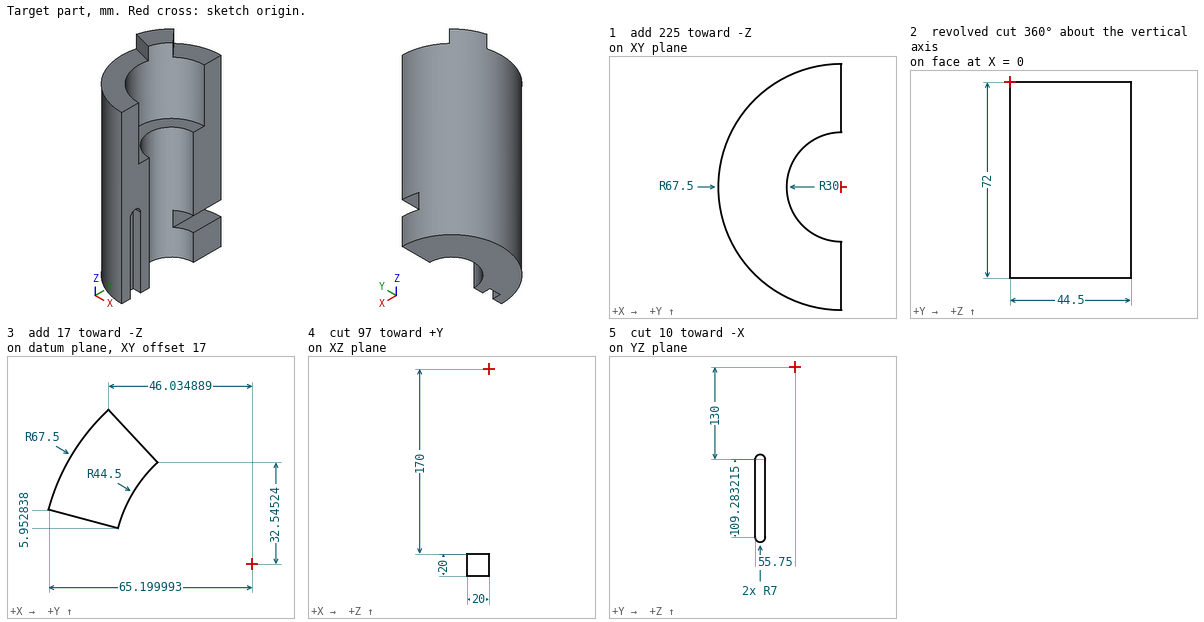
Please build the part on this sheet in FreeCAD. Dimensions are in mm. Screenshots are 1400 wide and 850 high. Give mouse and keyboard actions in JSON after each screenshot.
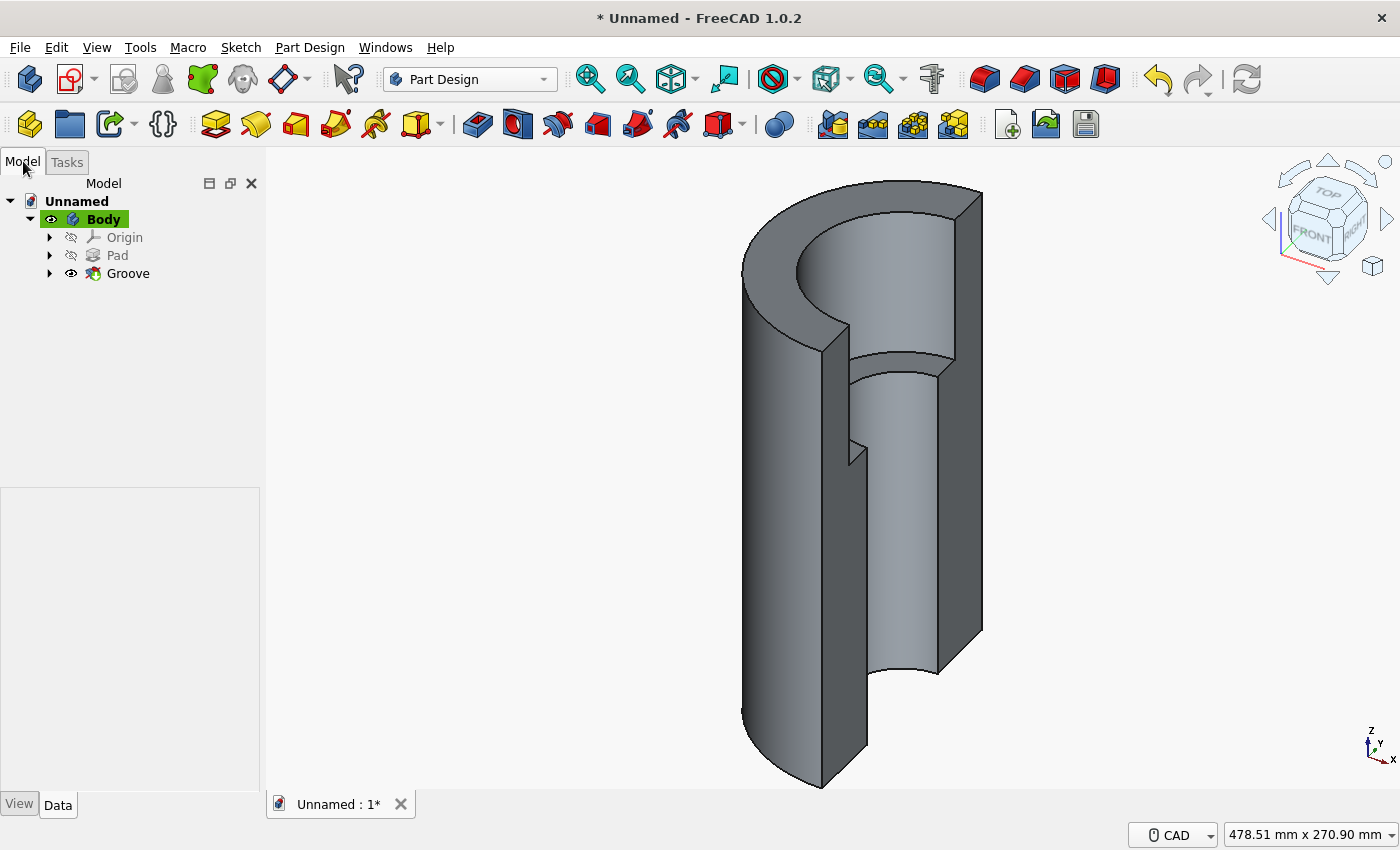
{"action": "left_click", "coordinate": [50, 237]}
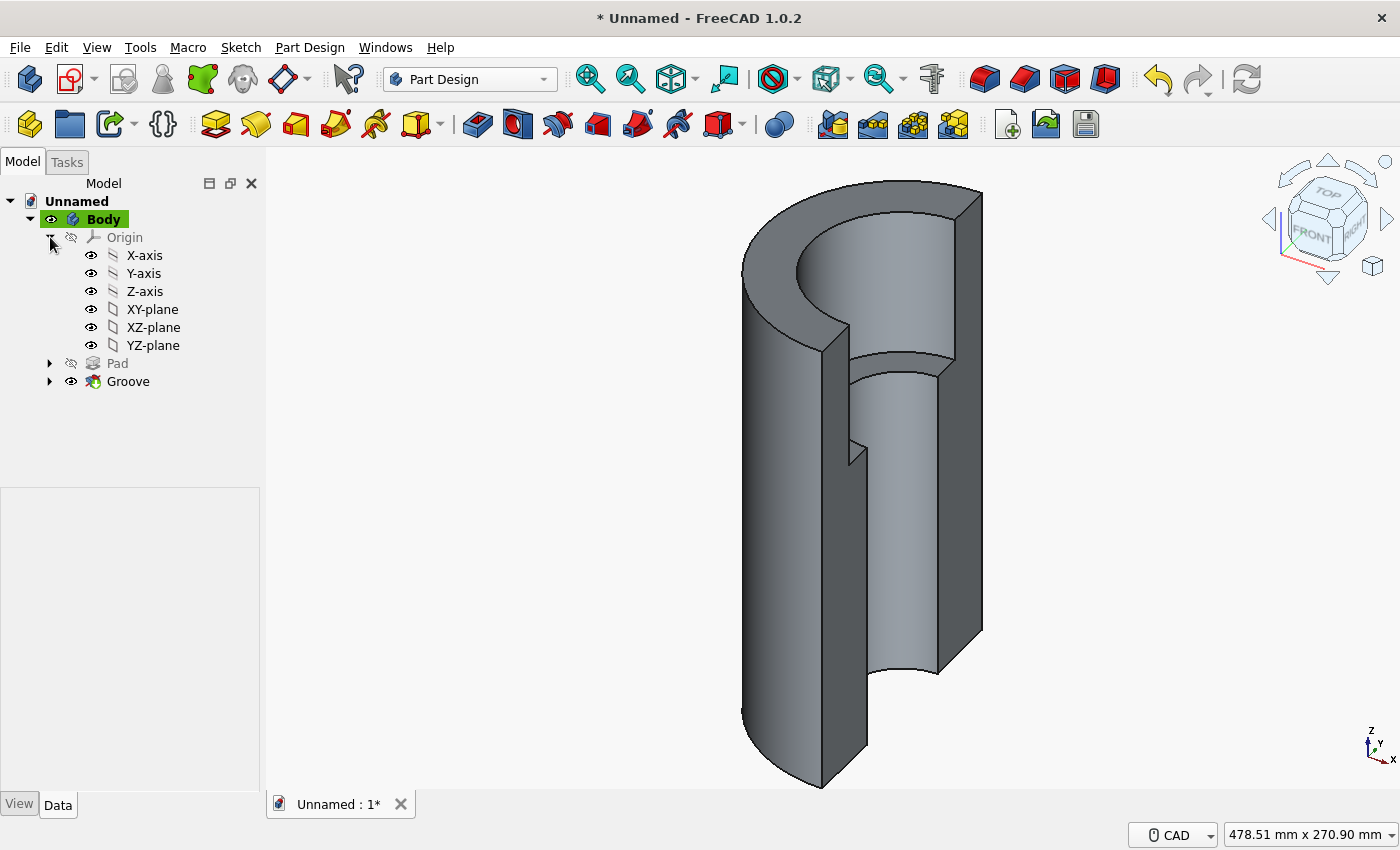
{"action": "left_click", "coordinate": [136, 309]}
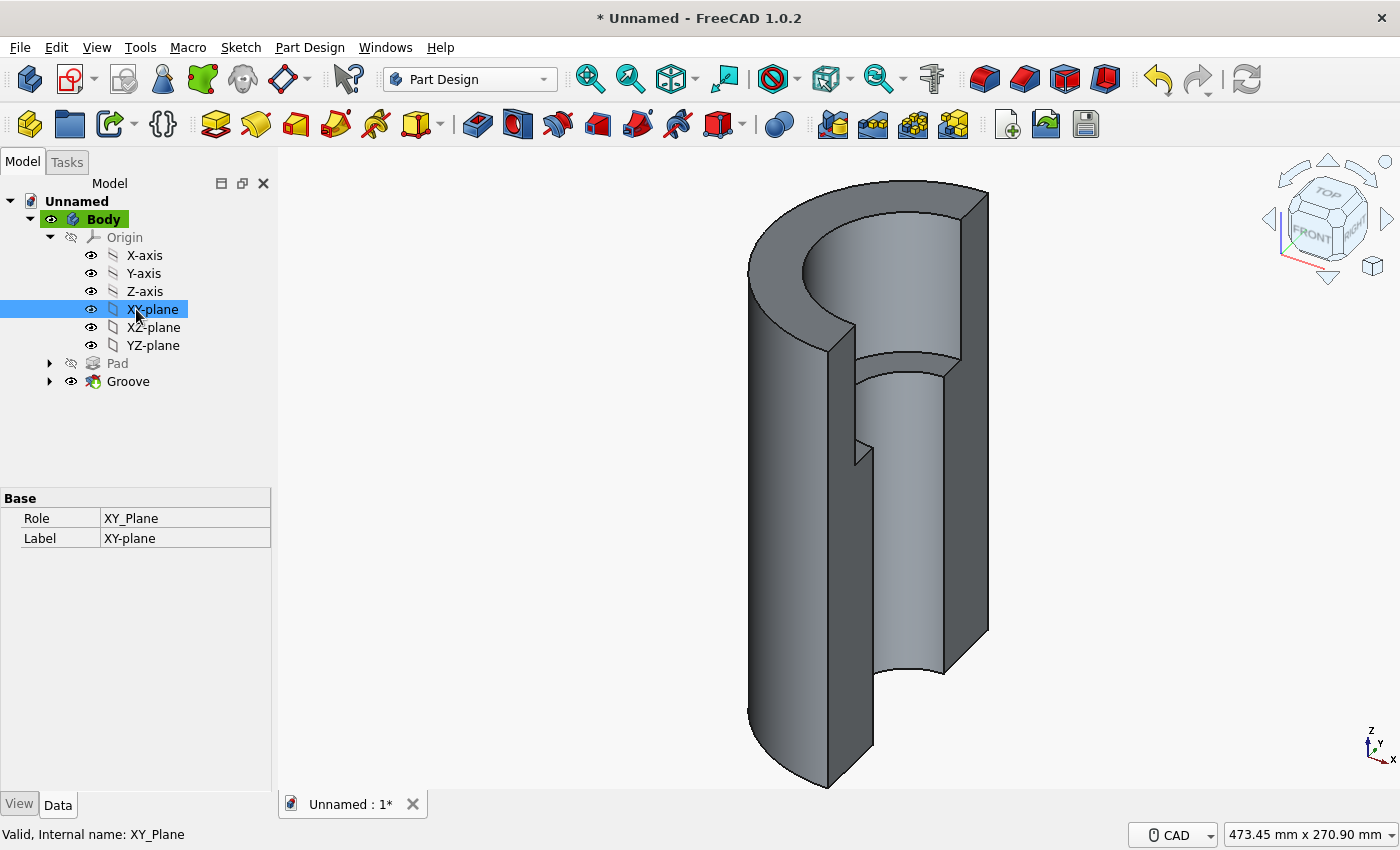
{"action": "left_click", "coordinate": [284, 80]}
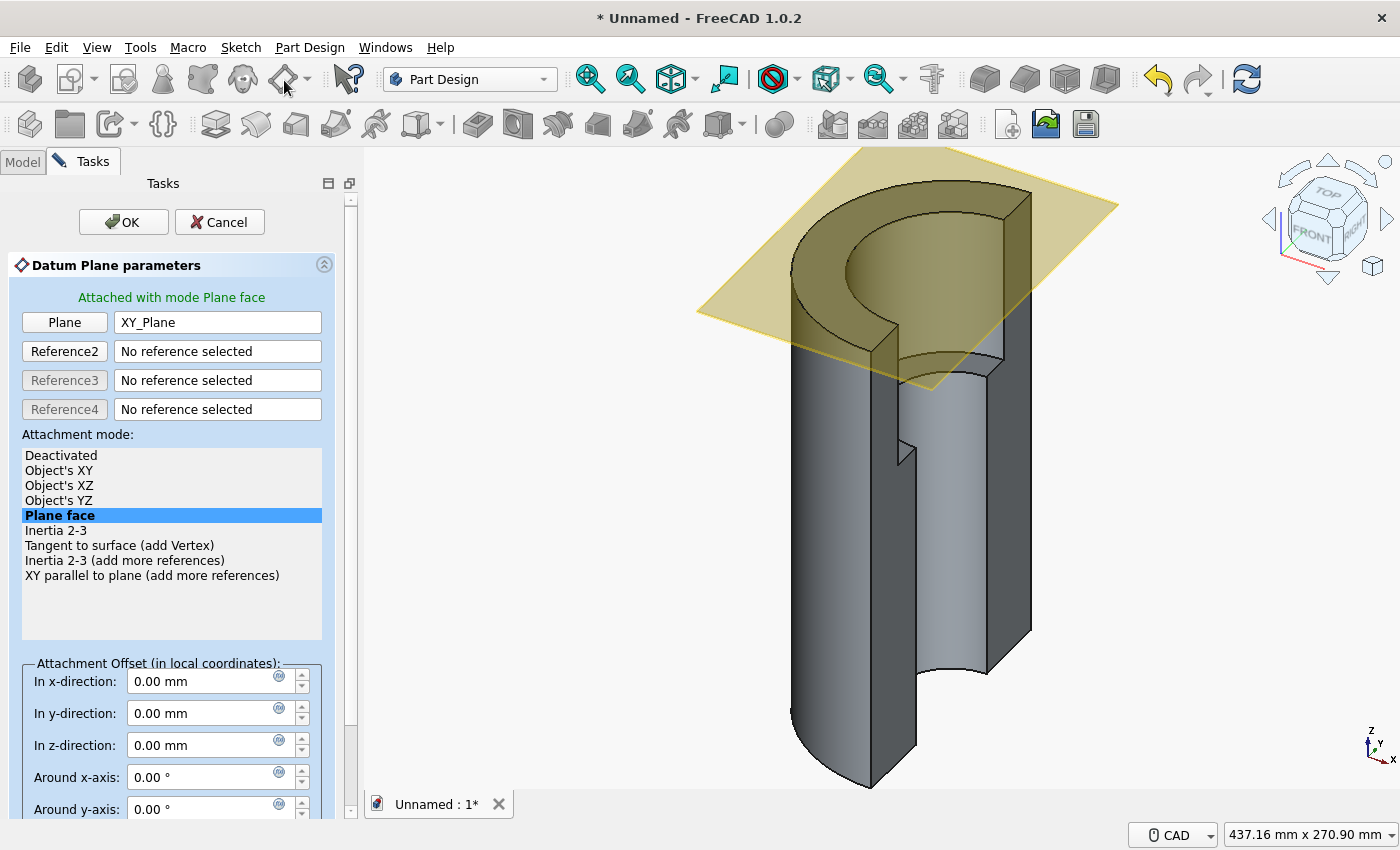
{"action": "triple_click", "coordinate": [210, 745]}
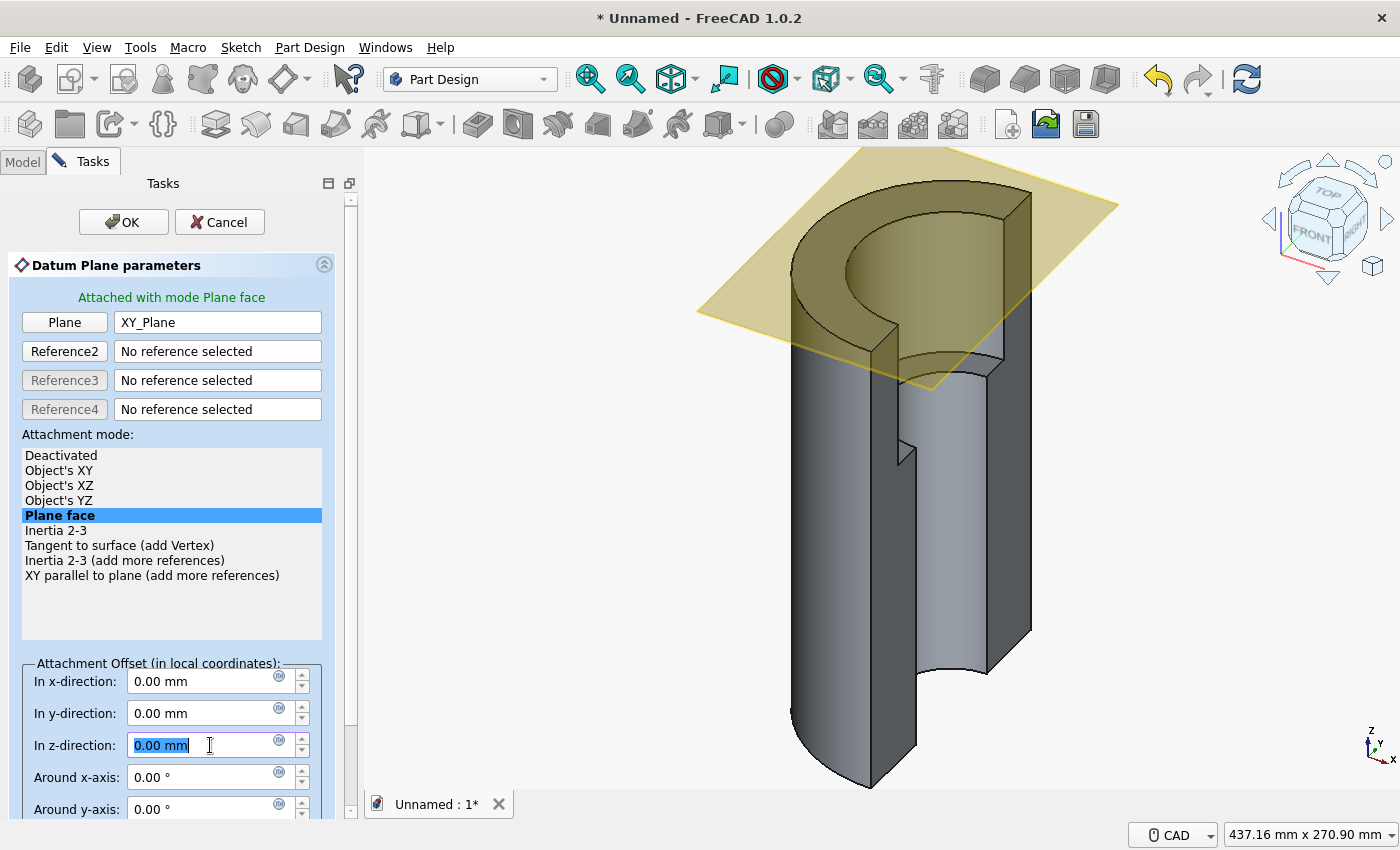
{"action": "type", "text": "17"}
{"action": "key", "text": "Tab"}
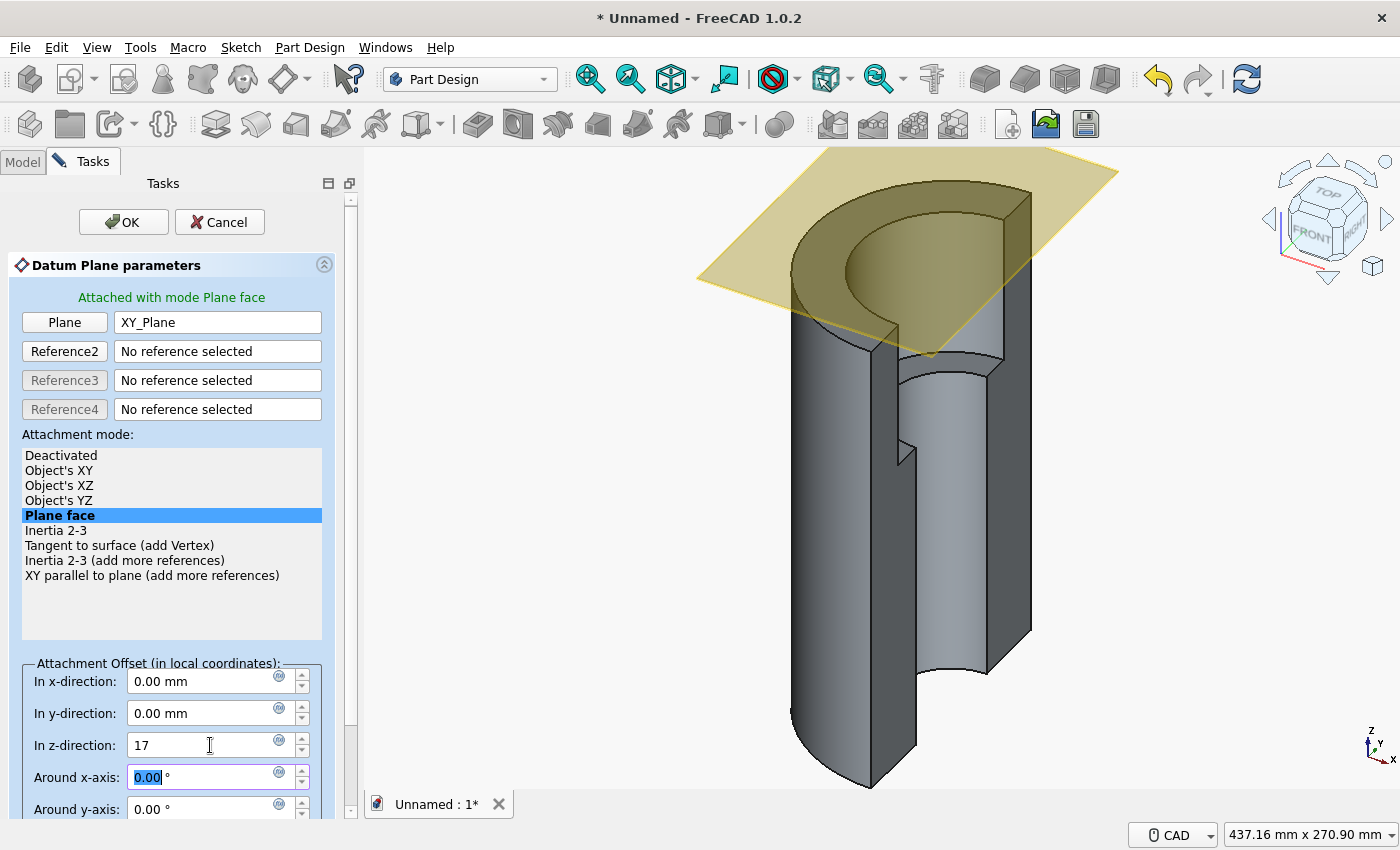
{"action": "left_click", "coordinate": [124, 222]}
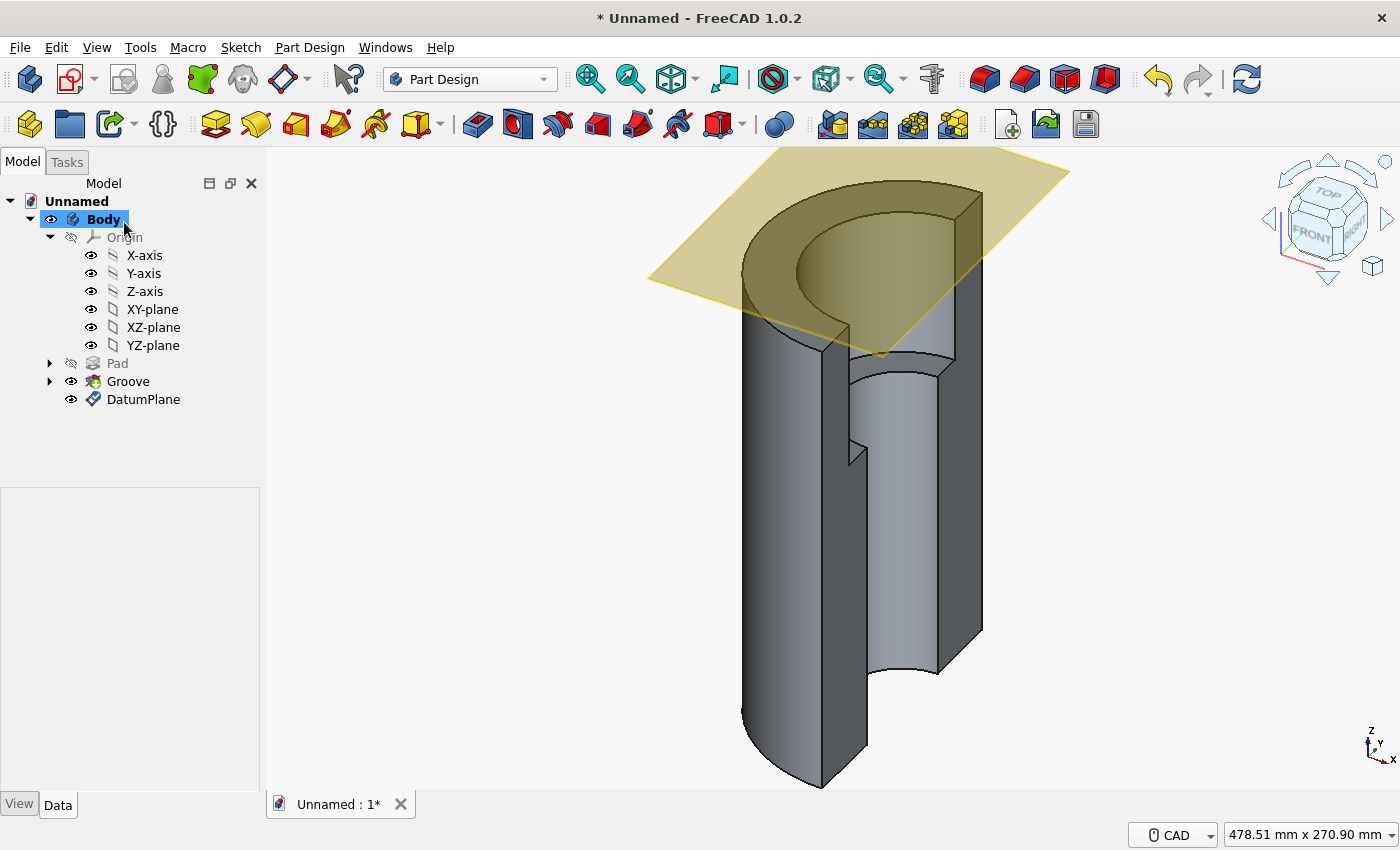
{"action": "left_click", "coordinate": [116, 399]}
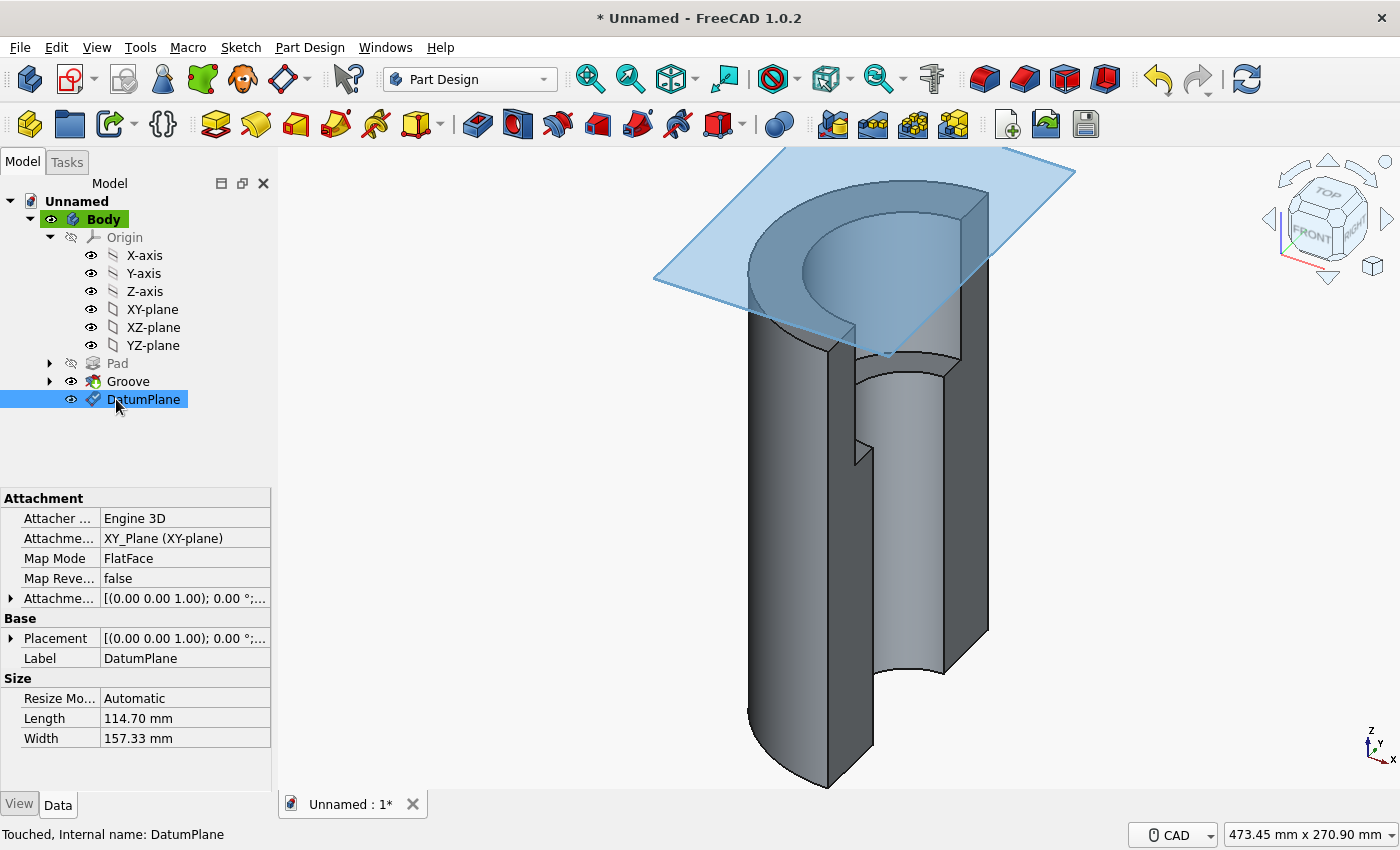
{"action": "left_click", "coordinate": [70, 80]}